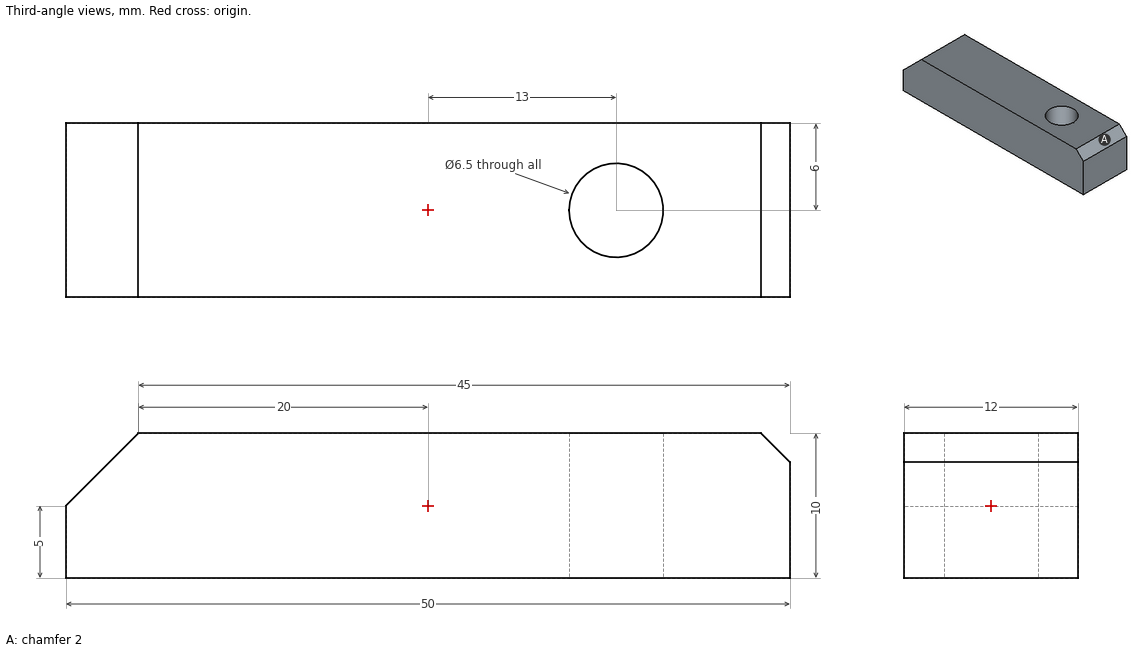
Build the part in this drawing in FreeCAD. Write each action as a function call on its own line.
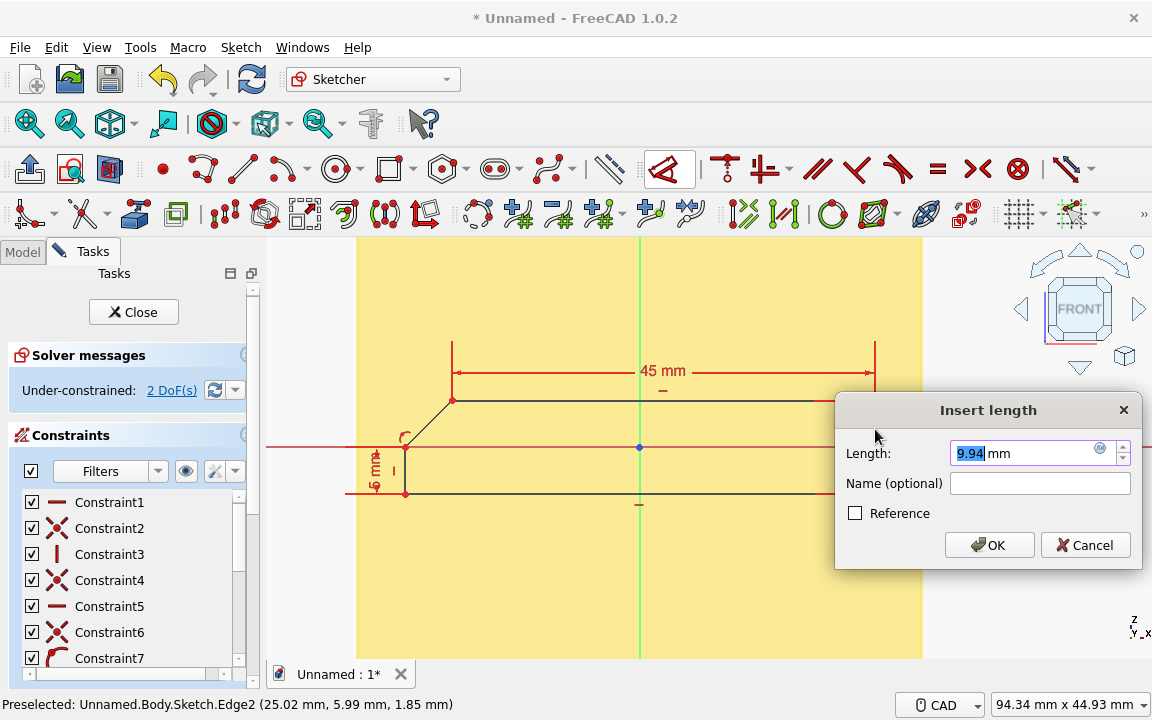
text(10)
key(Return)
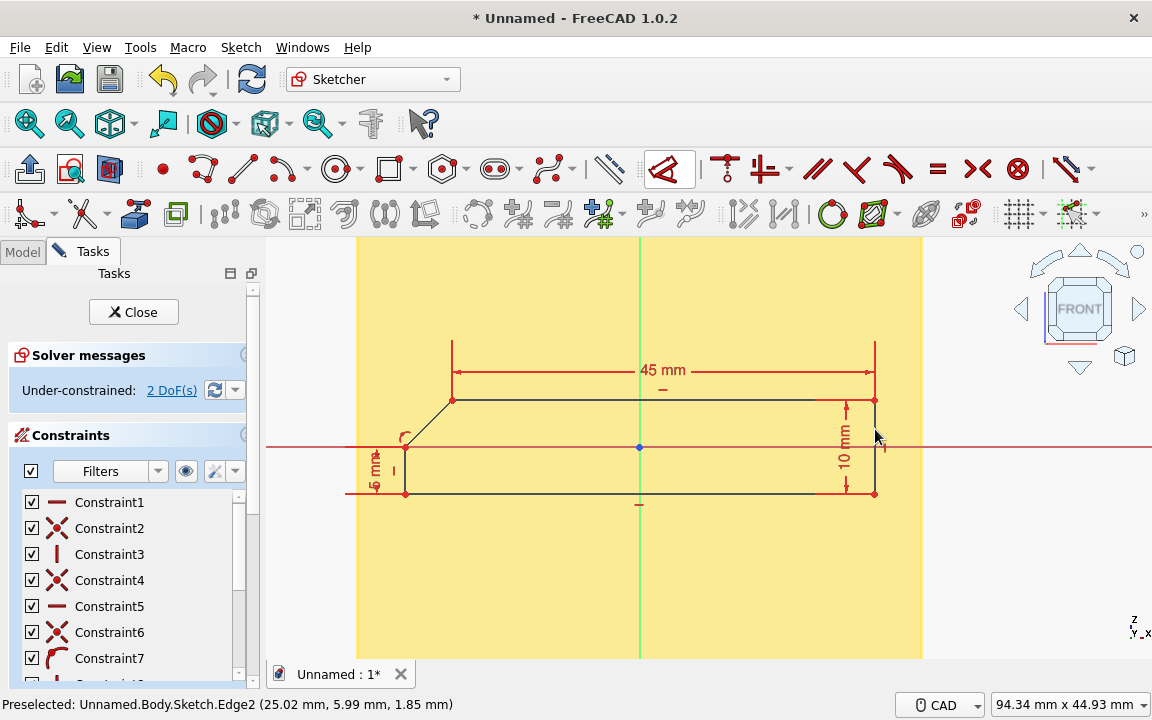
click(734, 494)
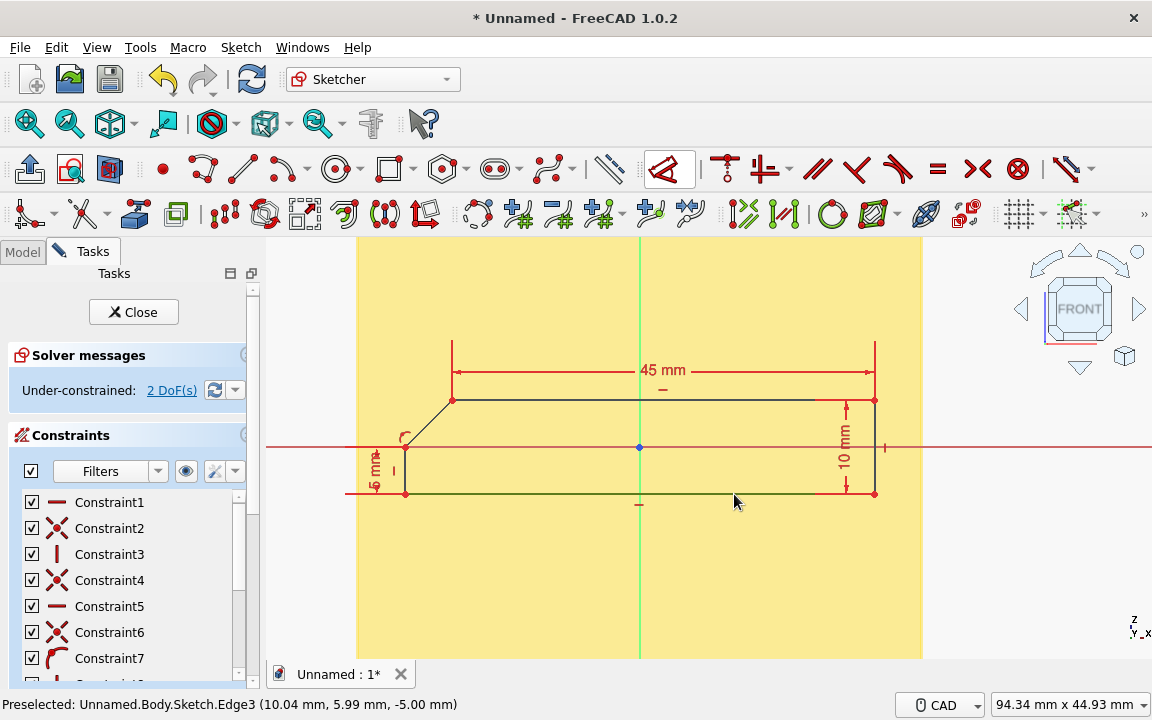
key(l)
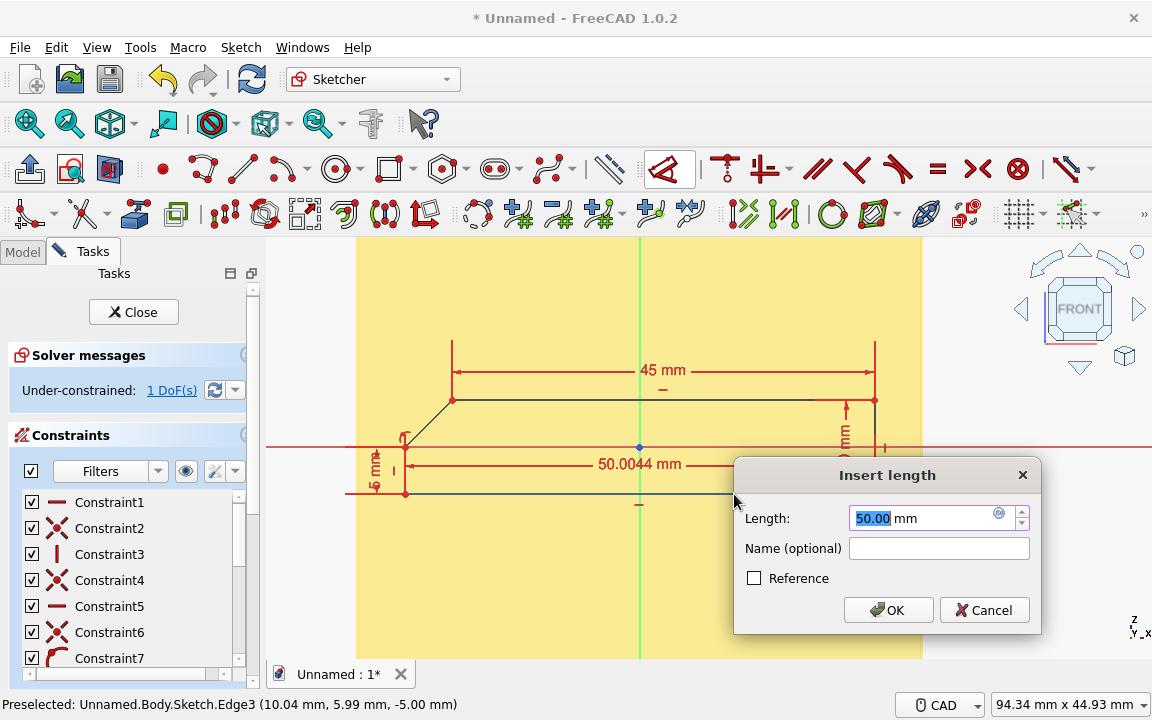
text(50)
key(Return)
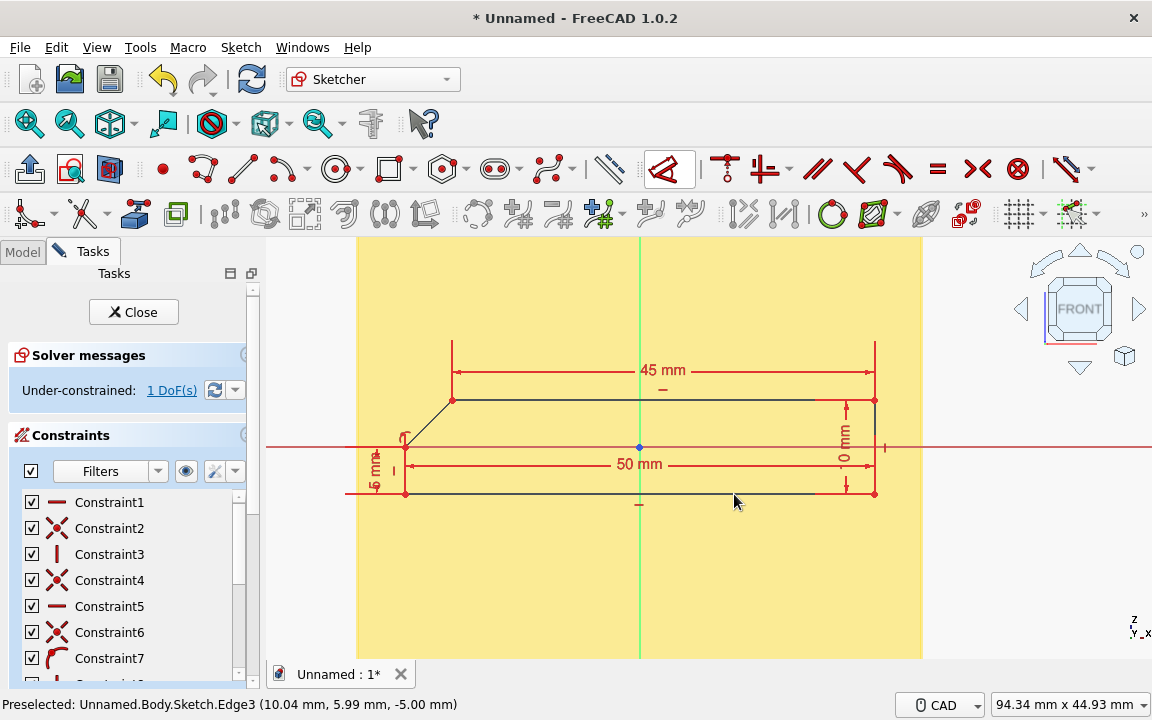
click(452, 400)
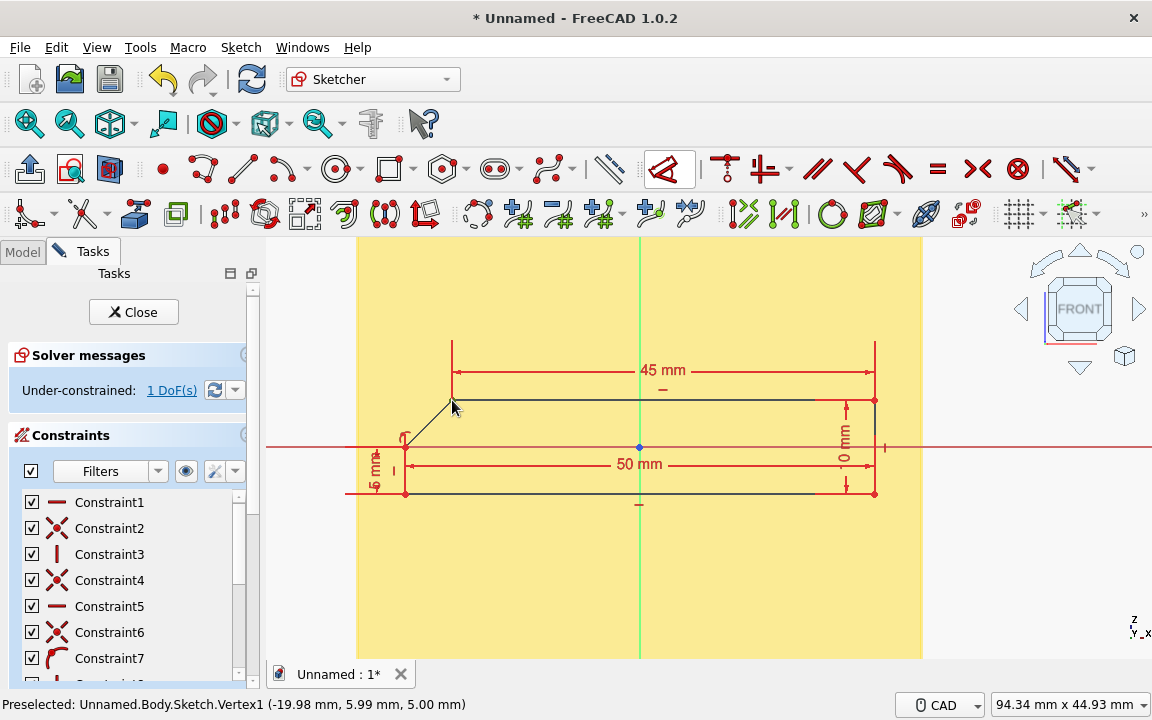
click(690, 170)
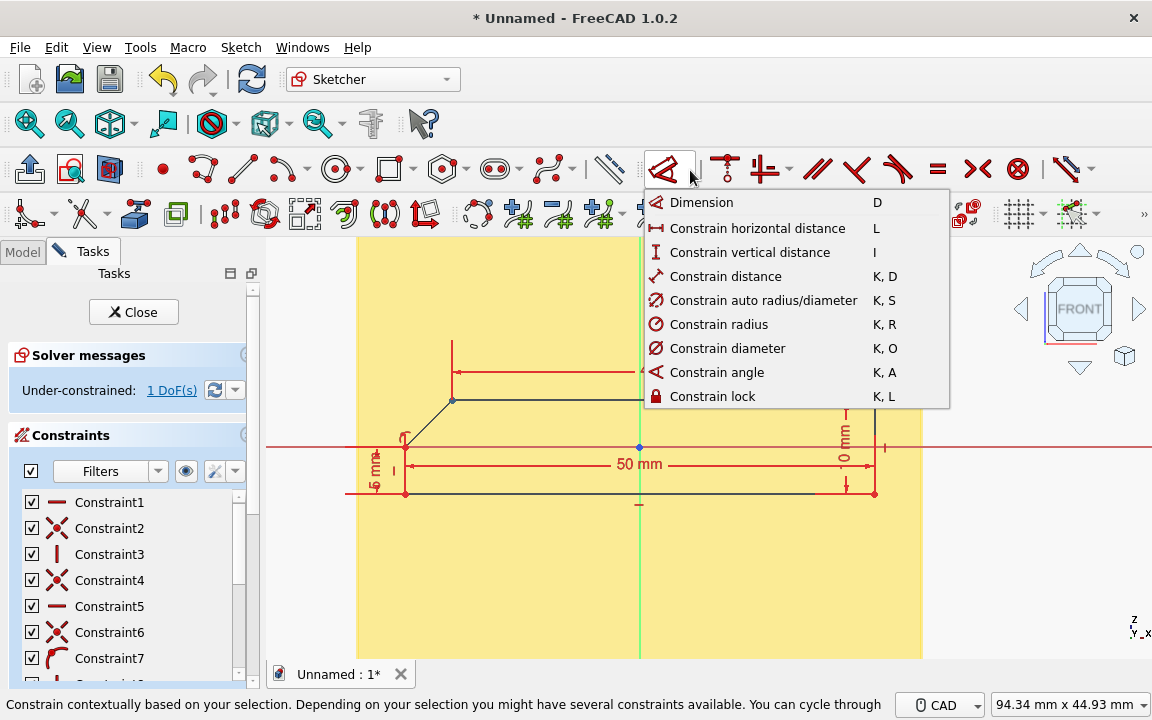
click(797, 228)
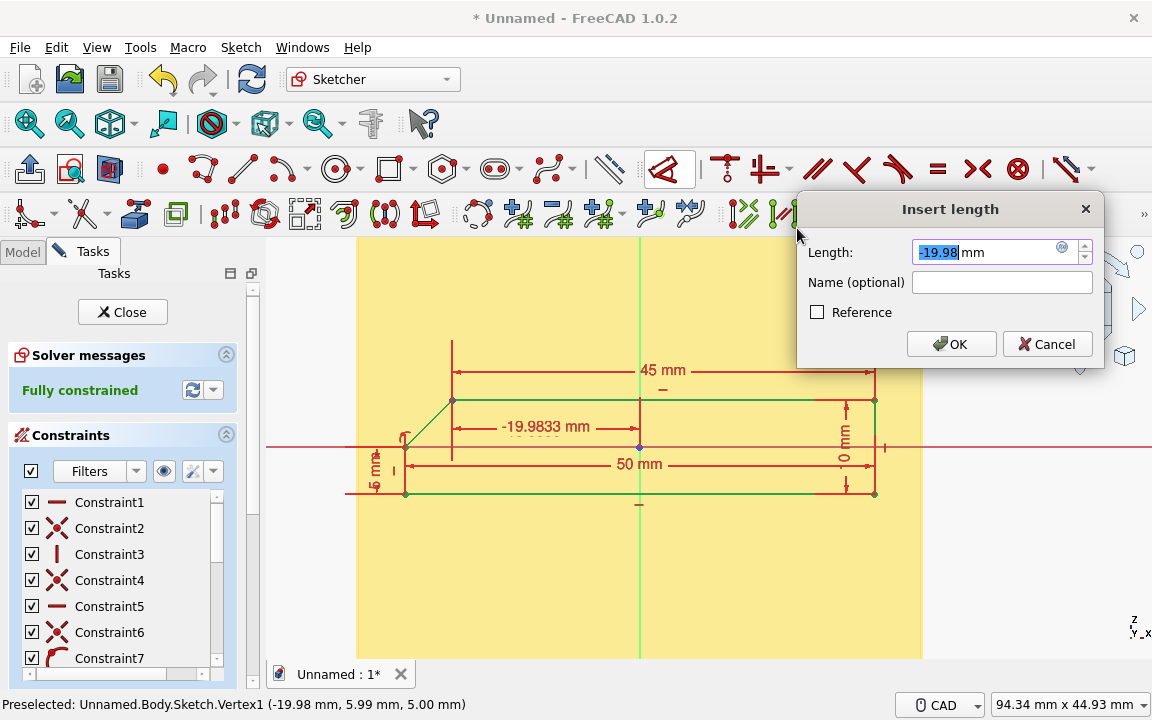
text(-20)
key(Return)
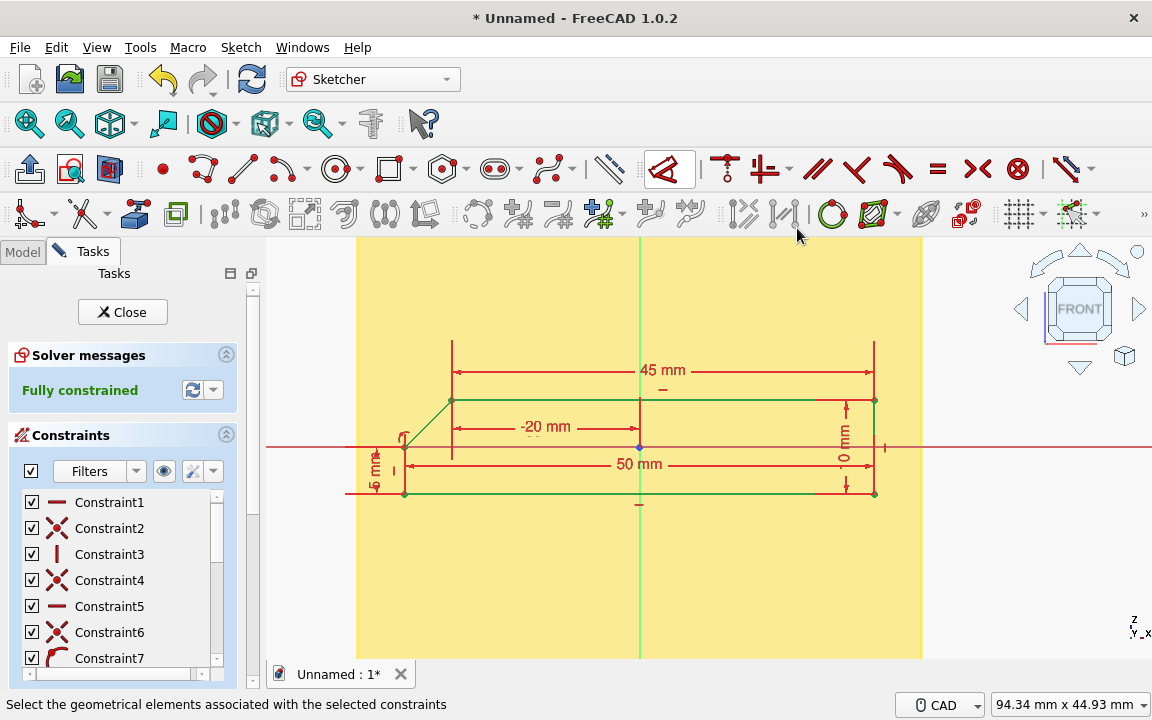
click(123, 312)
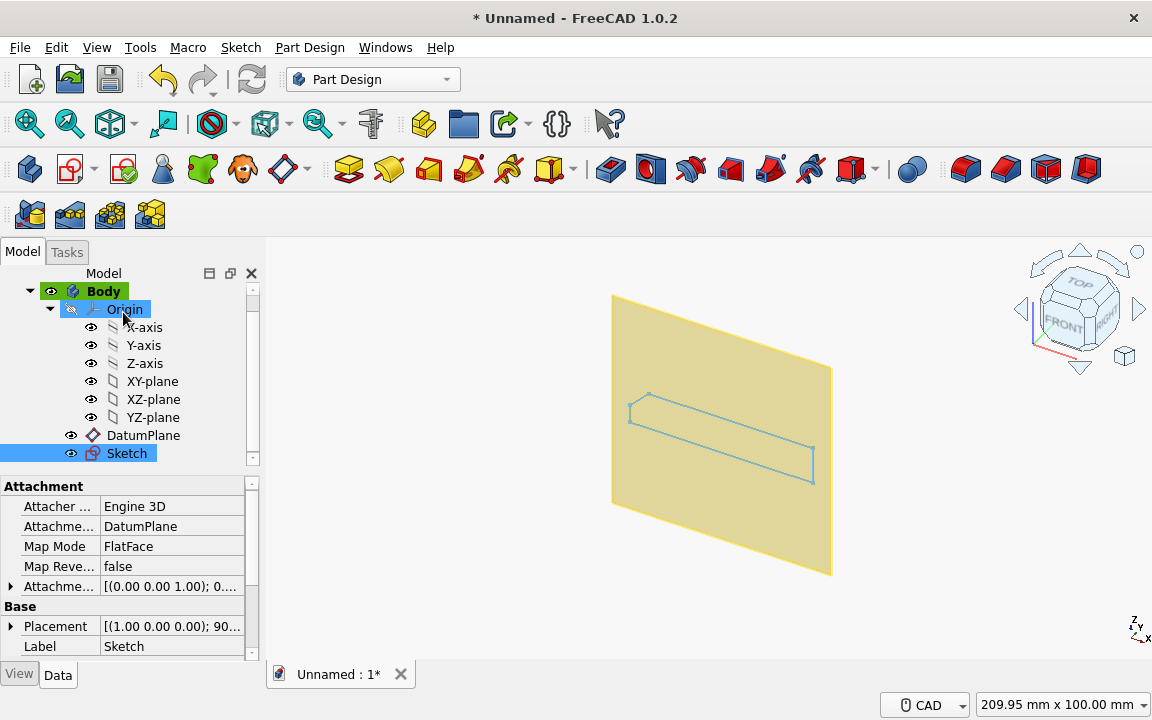
click(350, 170)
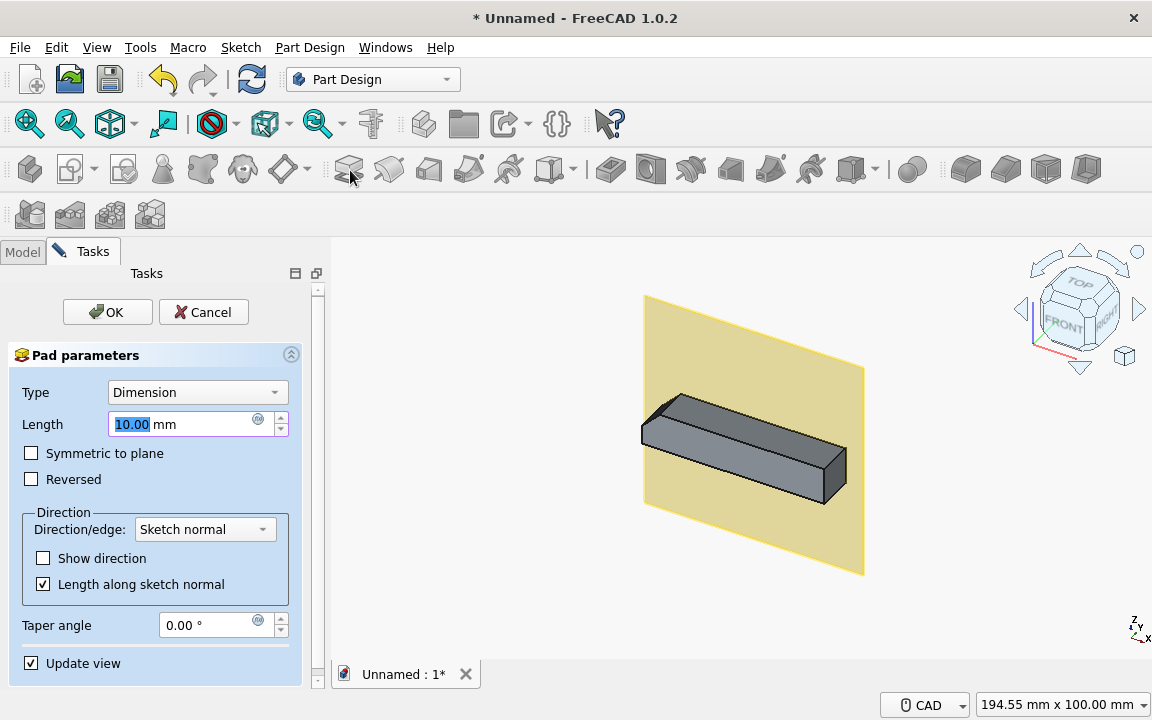
text(12)
key(Tab)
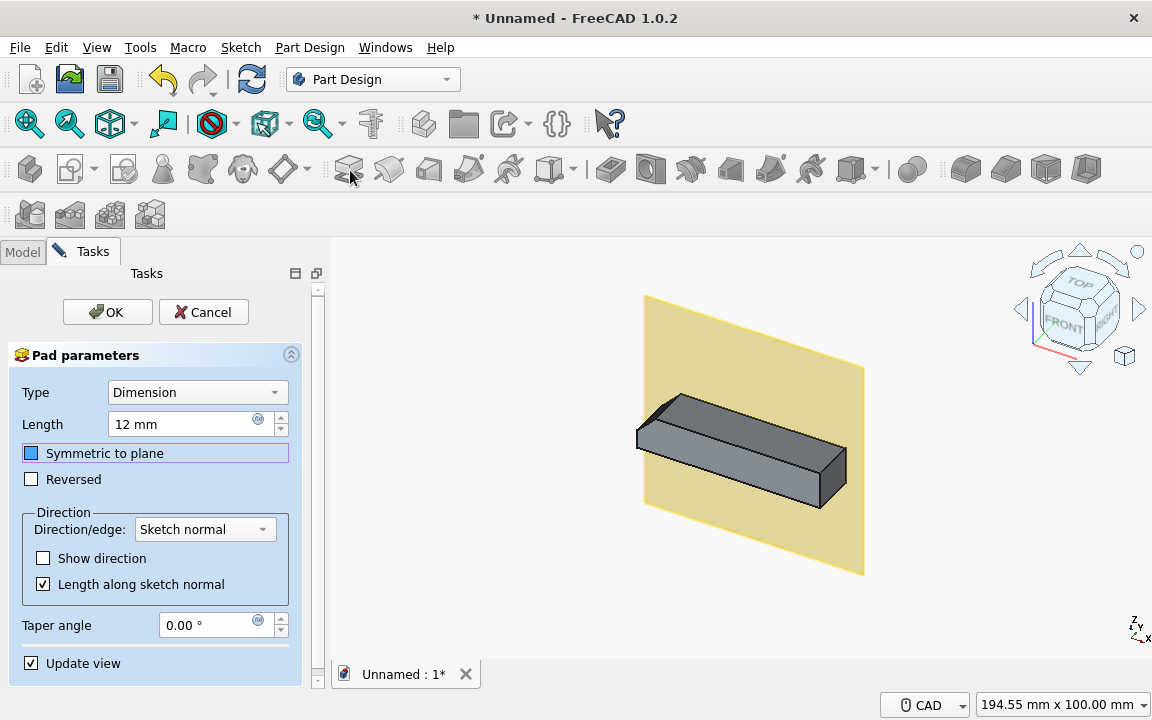
click(108, 312)